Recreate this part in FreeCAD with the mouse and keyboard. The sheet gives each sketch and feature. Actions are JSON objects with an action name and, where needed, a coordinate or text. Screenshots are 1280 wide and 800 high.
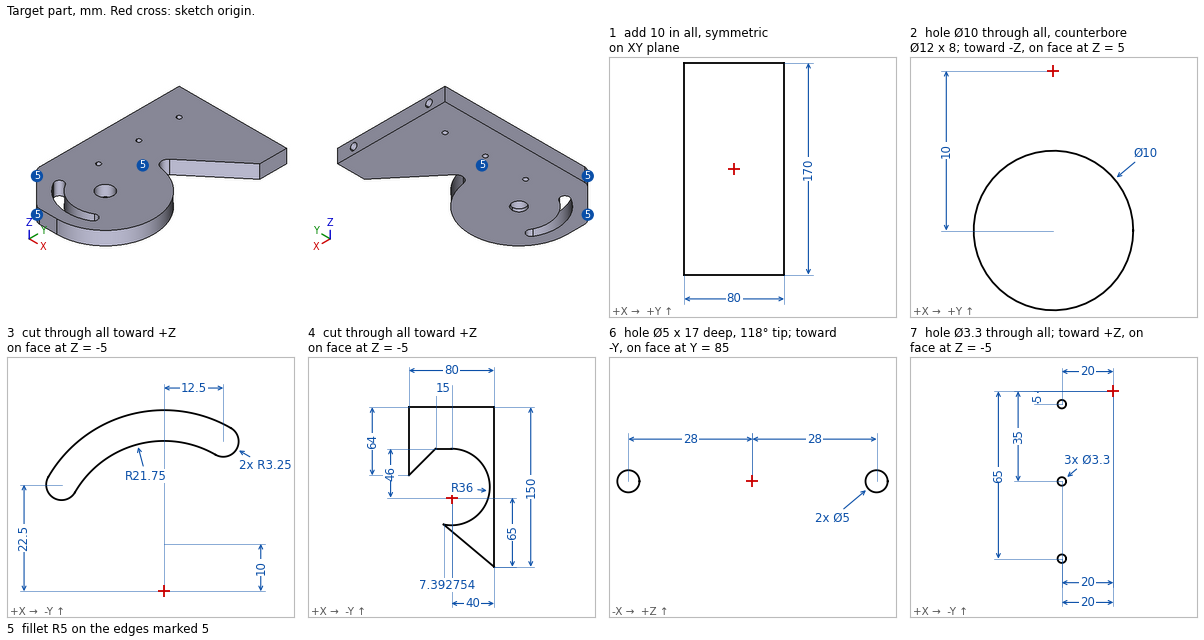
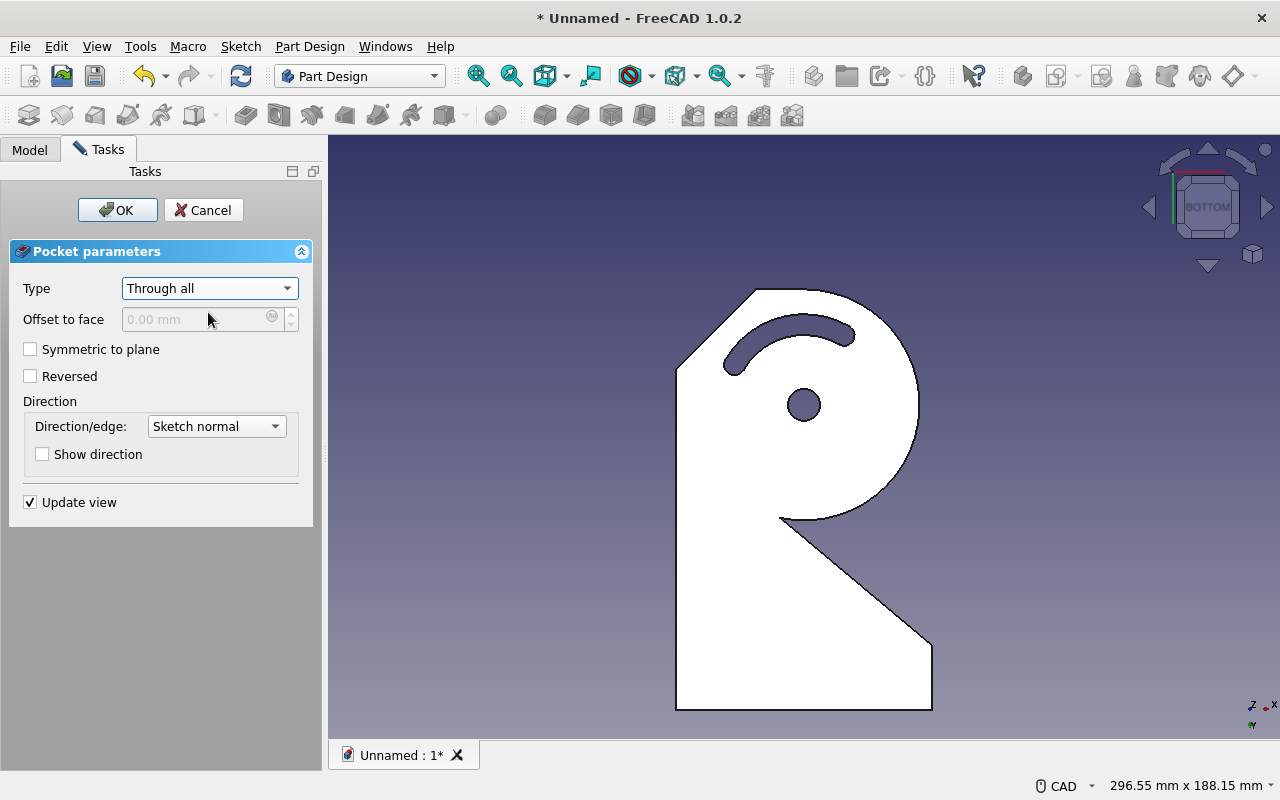
{"action": "left_click", "coordinate": [118, 210]}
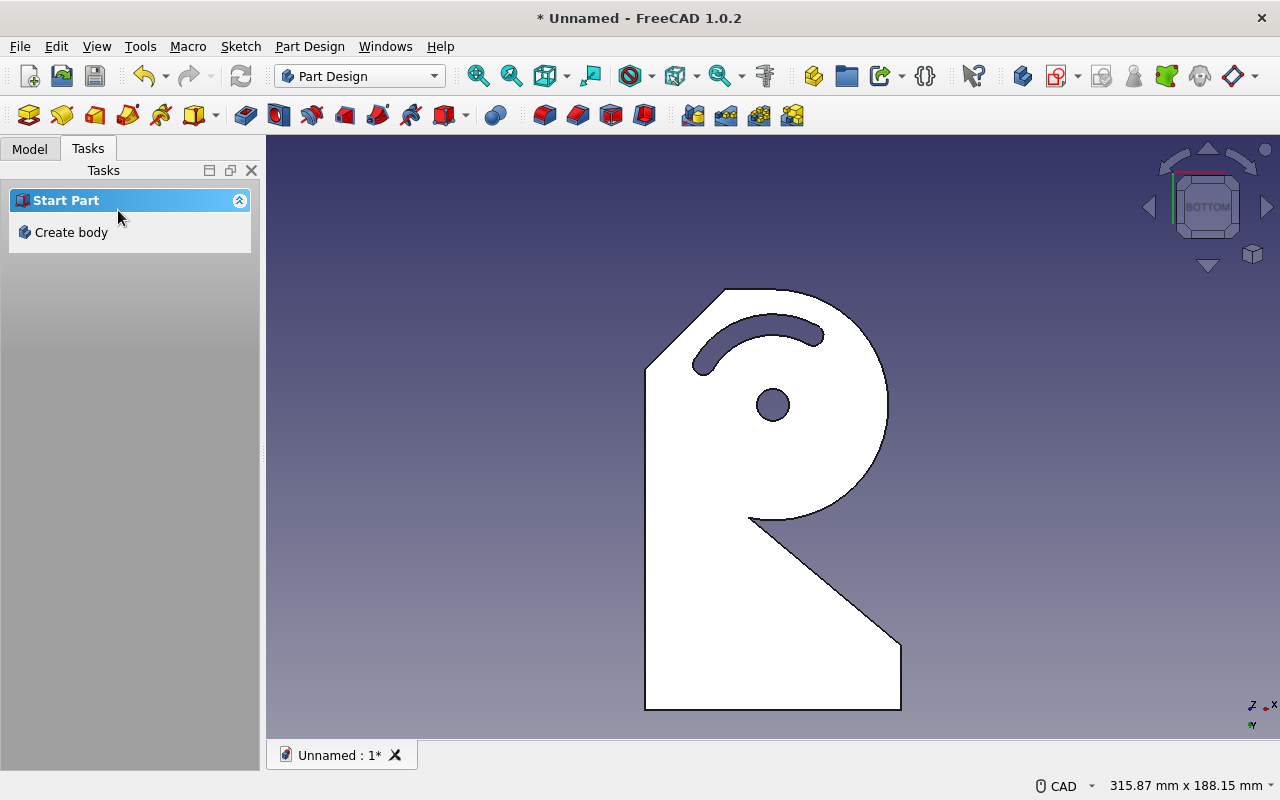
{"action": "key", "text": "0"}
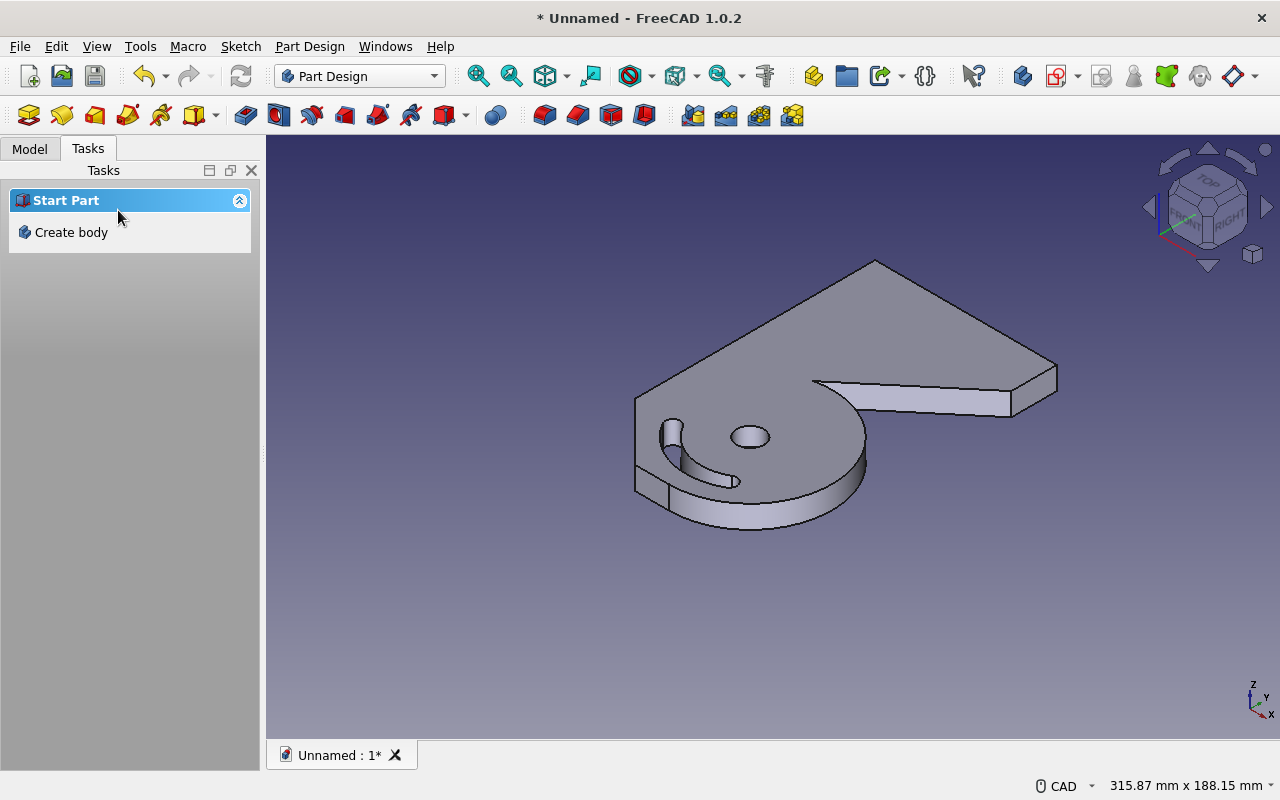
{"action": "key", "text": "2"}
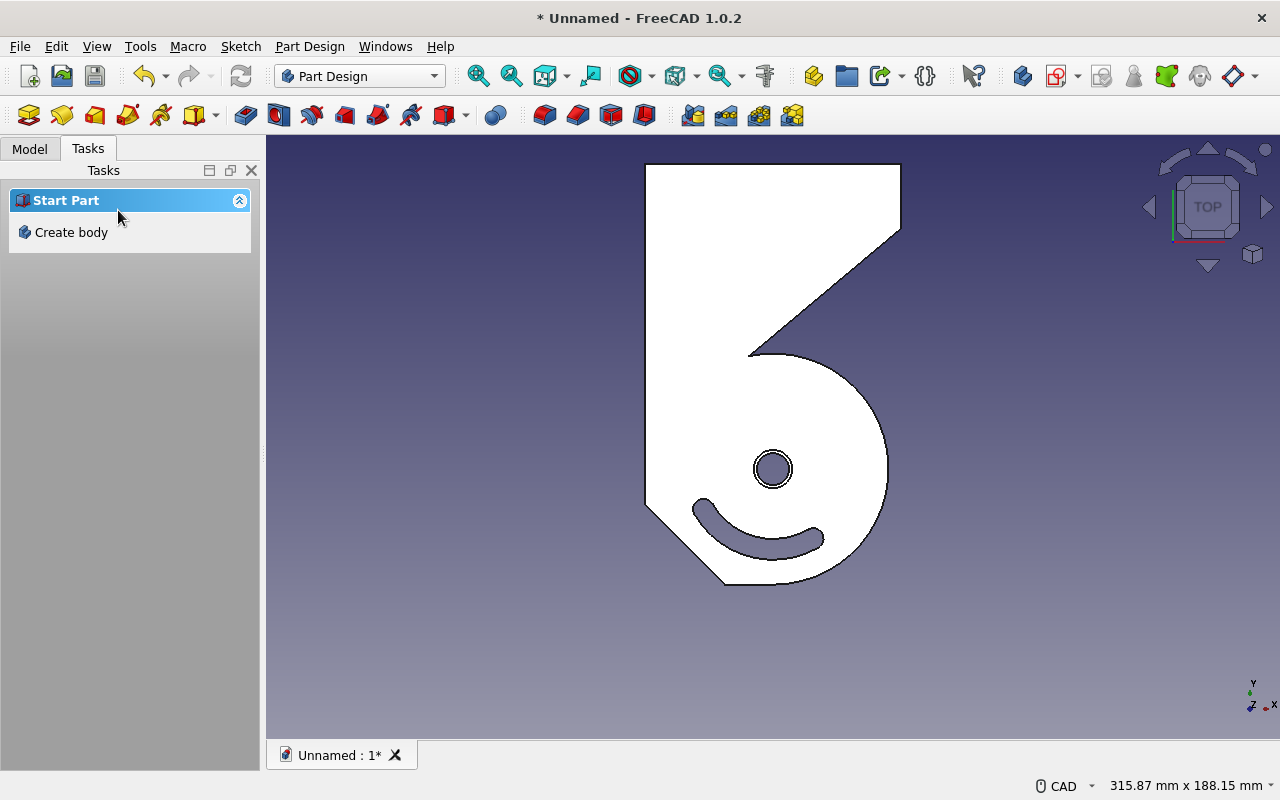
{"action": "key", "text": "1"}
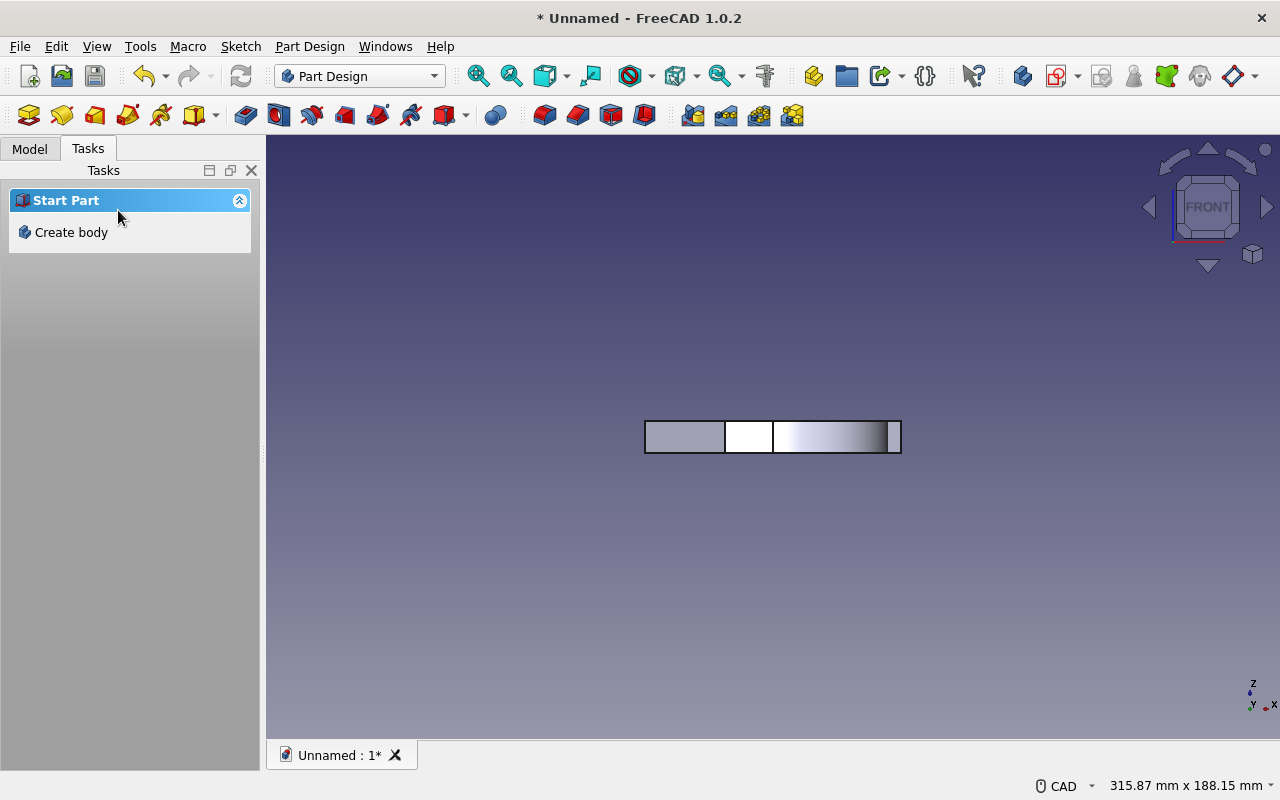
{"action": "left_click", "coordinate": [479, 76]}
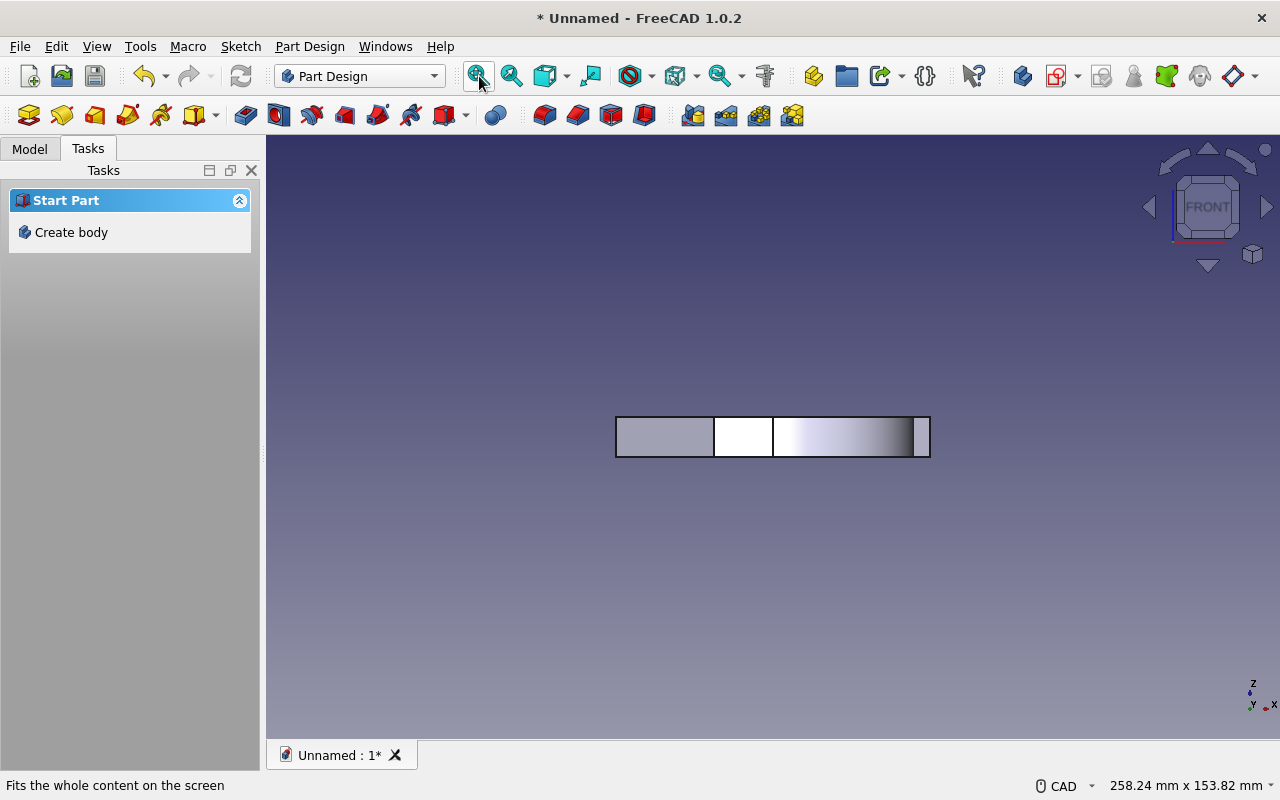
{"action": "left_click", "coordinate": [714, 436]}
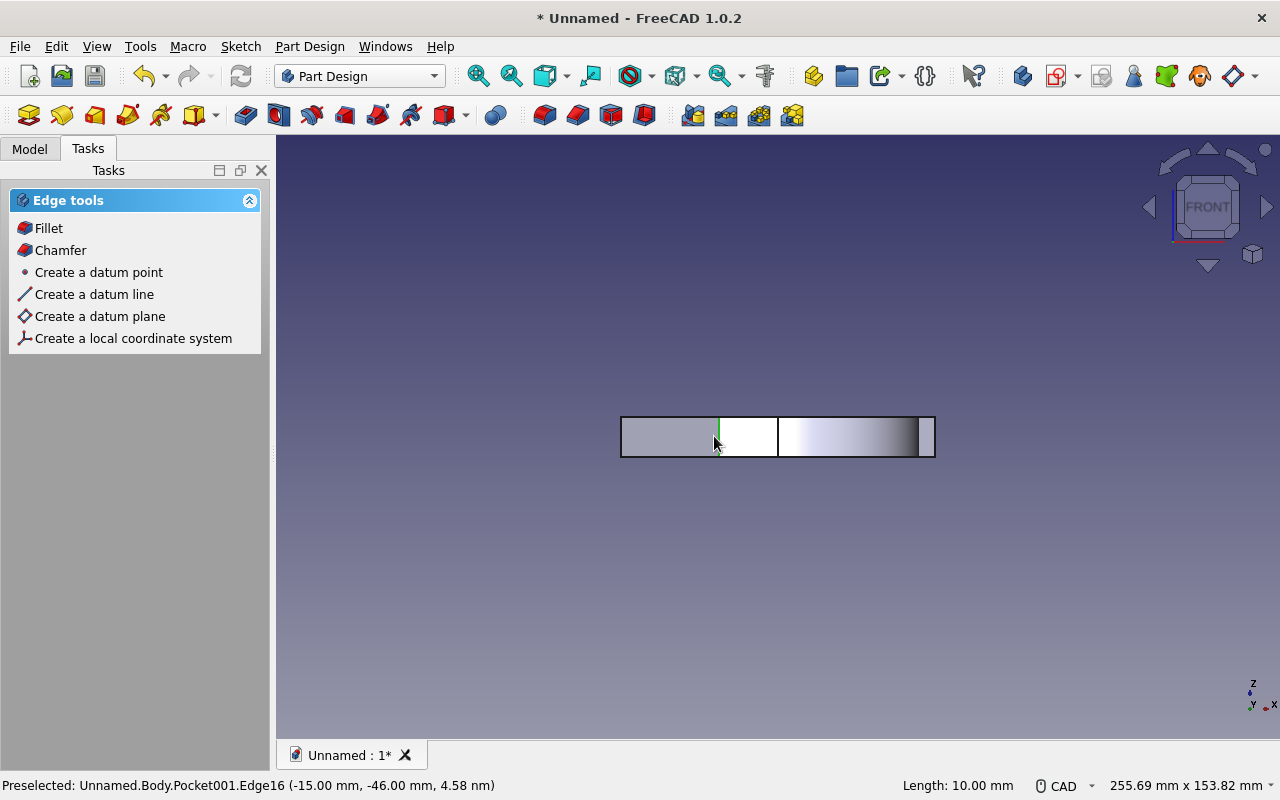
{"action": "key", "text": "3"}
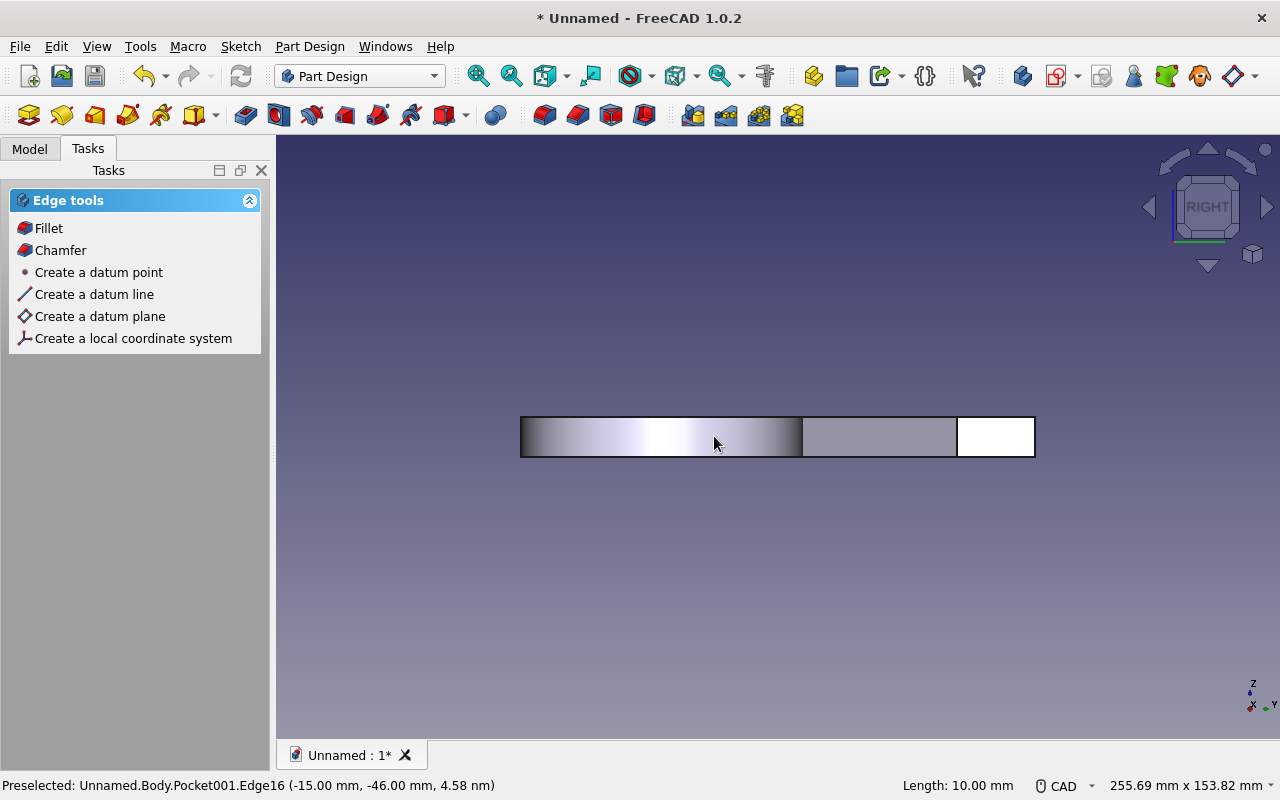
{"action": "key", "text": "5"}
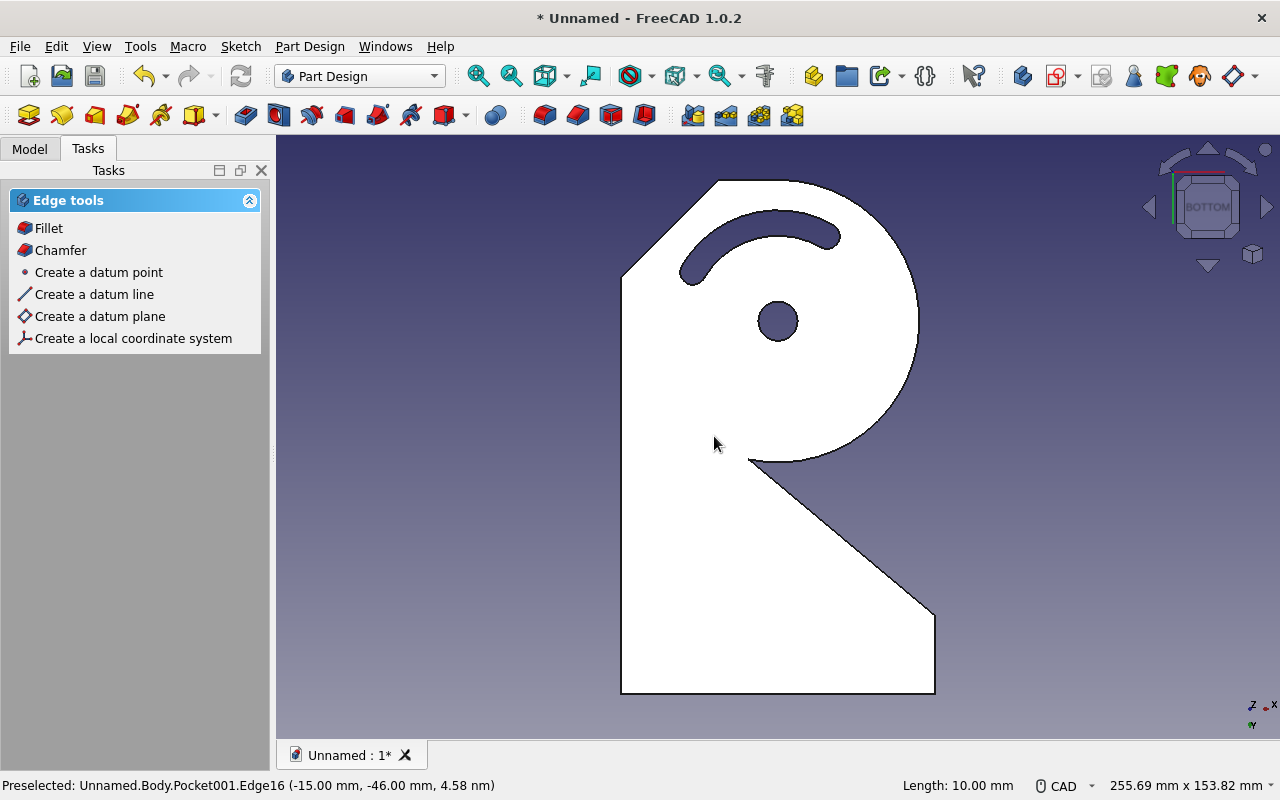
{"action": "key", "text": "4"}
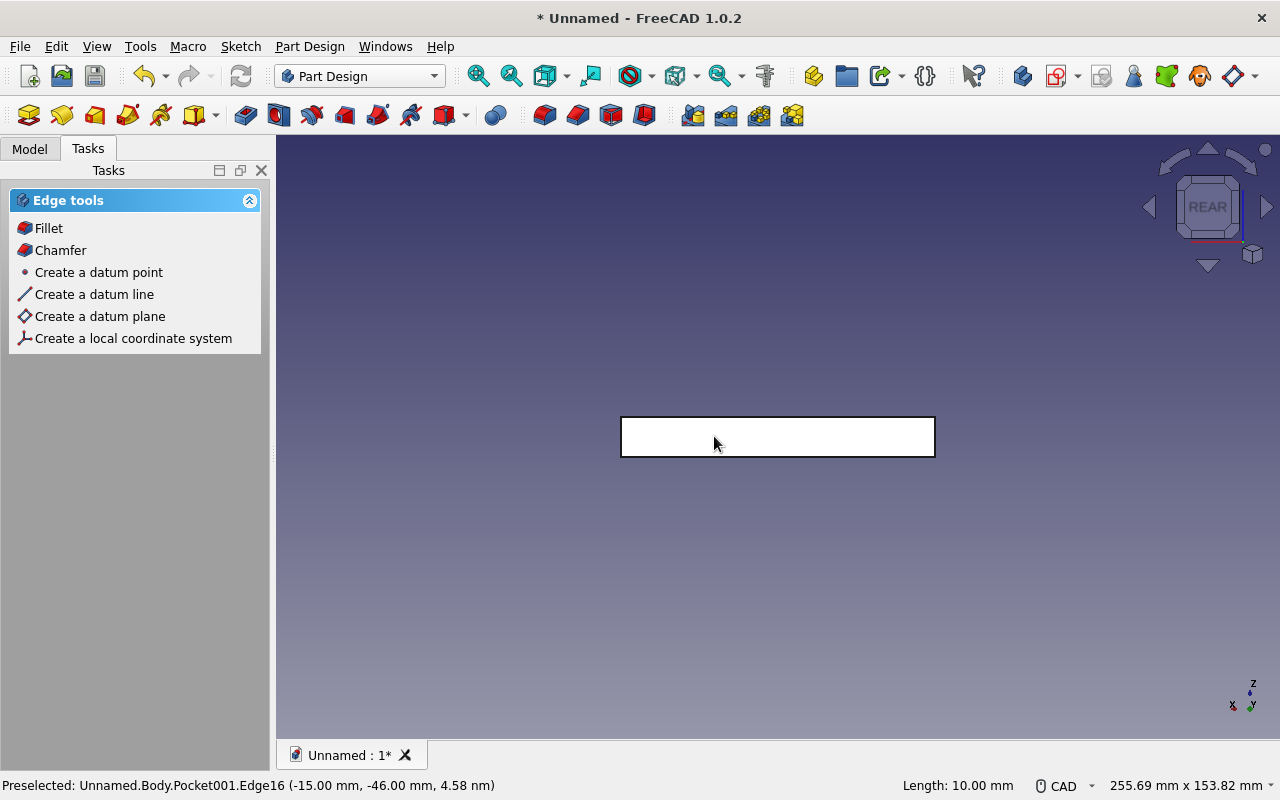
{"action": "key", "text": "v f"}